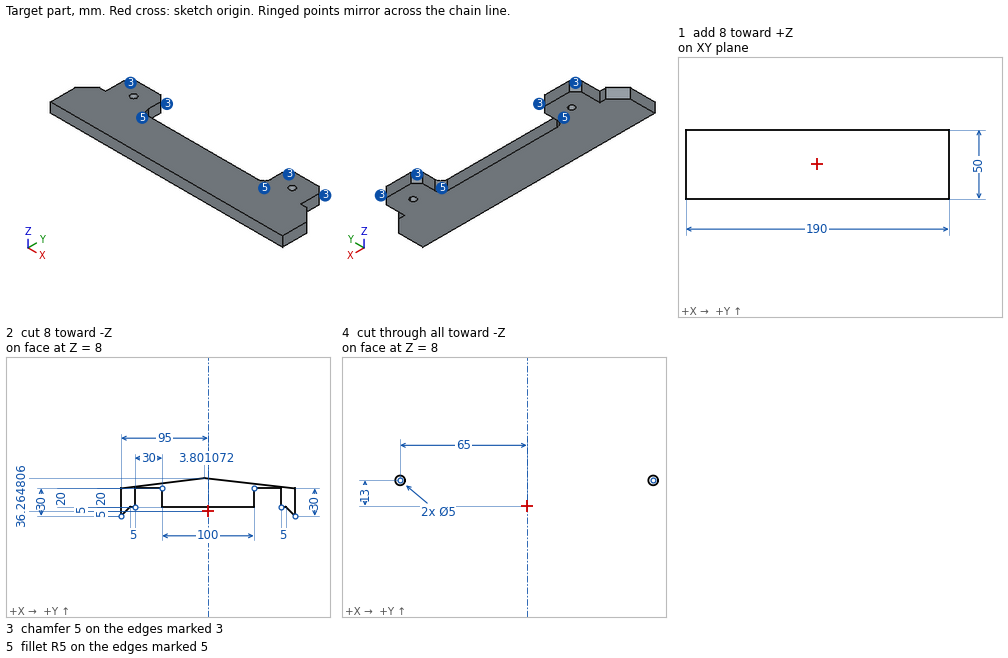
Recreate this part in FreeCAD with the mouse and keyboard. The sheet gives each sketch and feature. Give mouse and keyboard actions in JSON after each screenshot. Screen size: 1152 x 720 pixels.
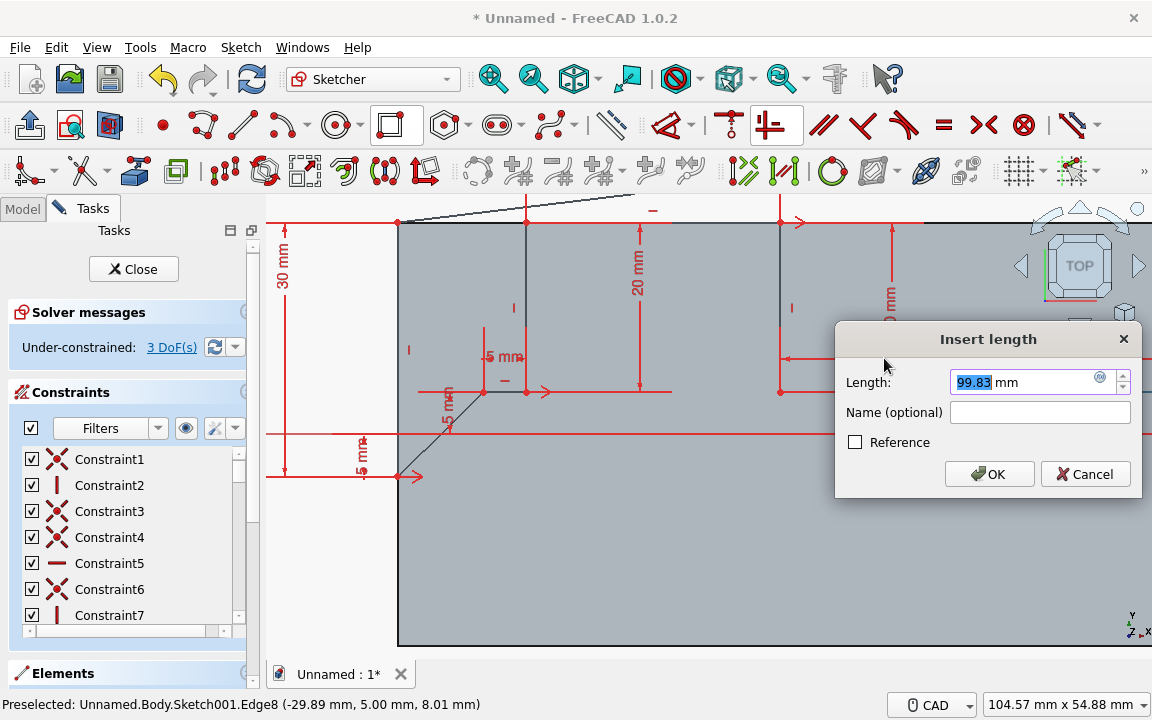
{"action": "type", "text": "100"}
{"action": "key", "text": "Return"}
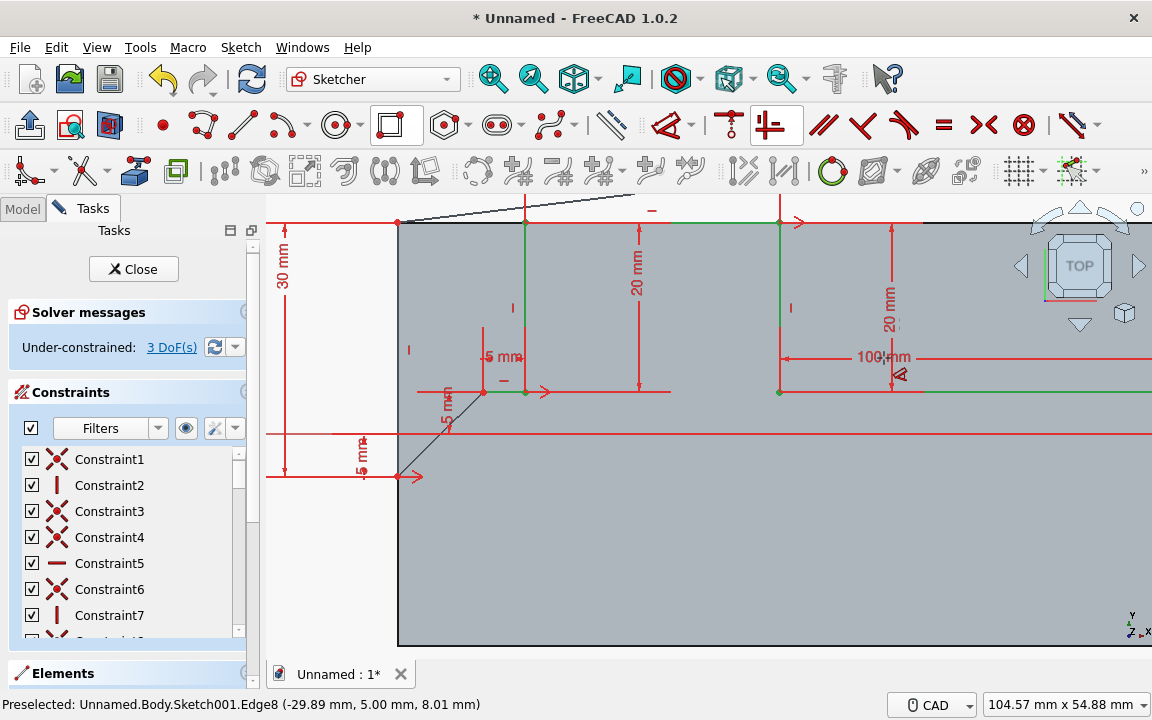
{"action": "left_click", "coordinate": [398, 223]}
{"action": "left_click", "coordinate": [692, 468]}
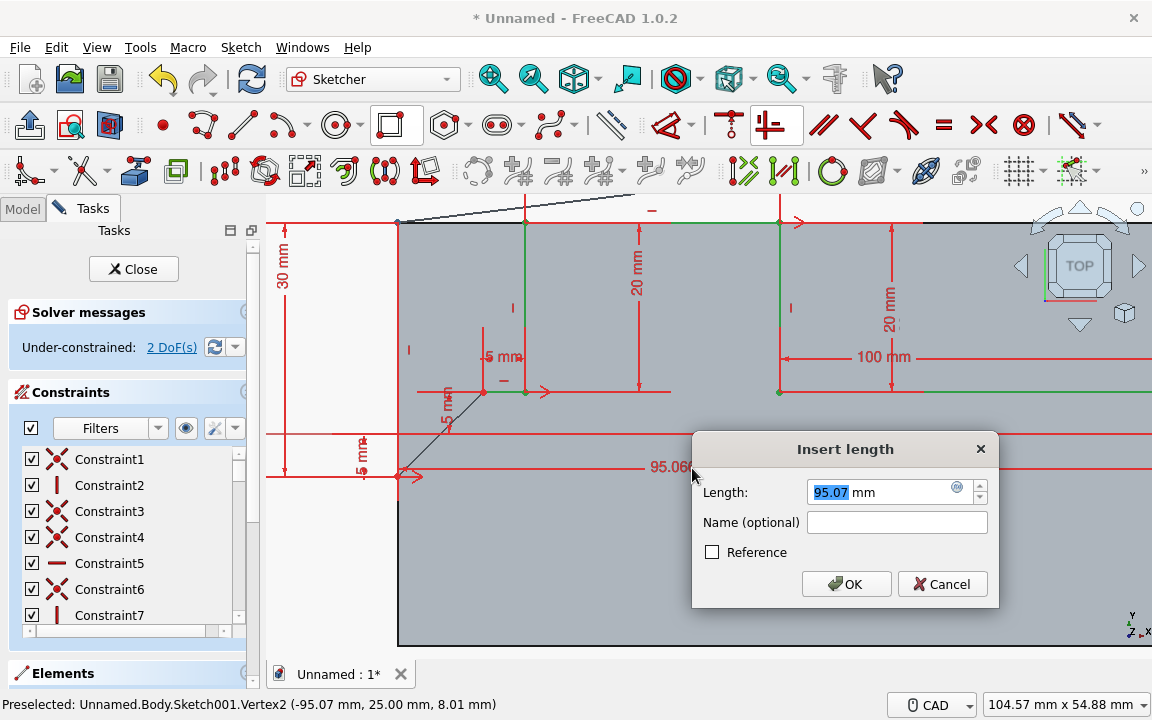
{"action": "type", "text": "95"}
{"action": "key", "text": "Return"}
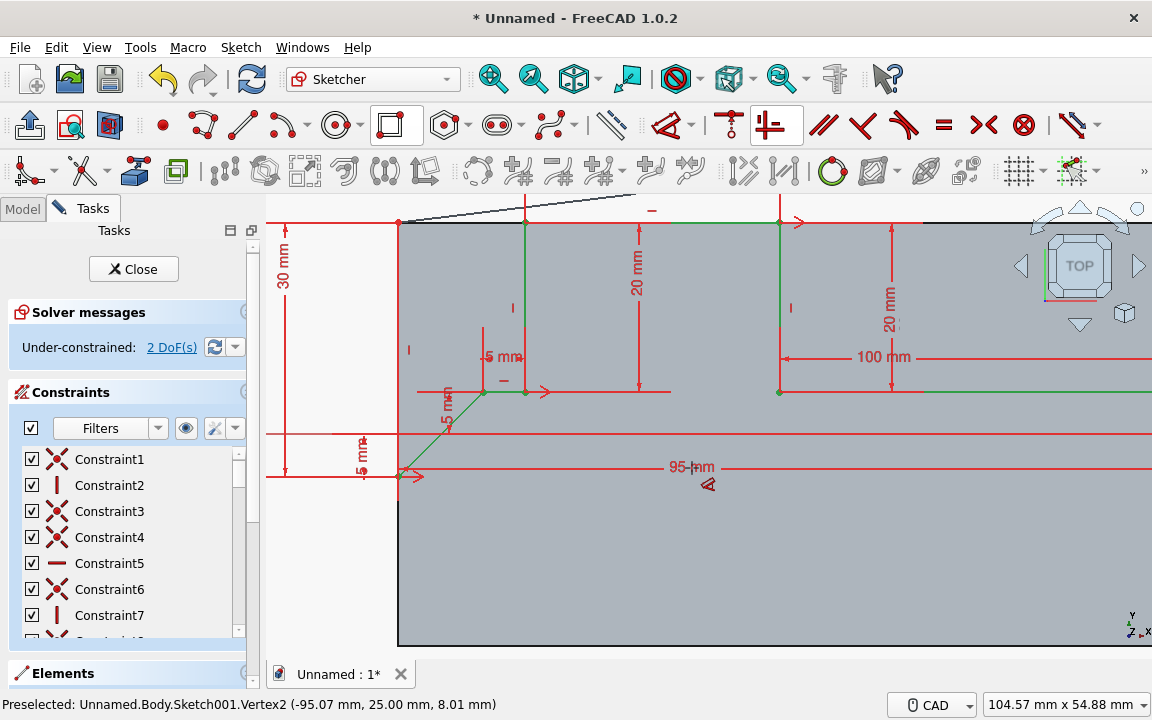
{"action": "scroll", "coordinate": [398, 480], "scroll_direction": "down", "scroll_amount": 6}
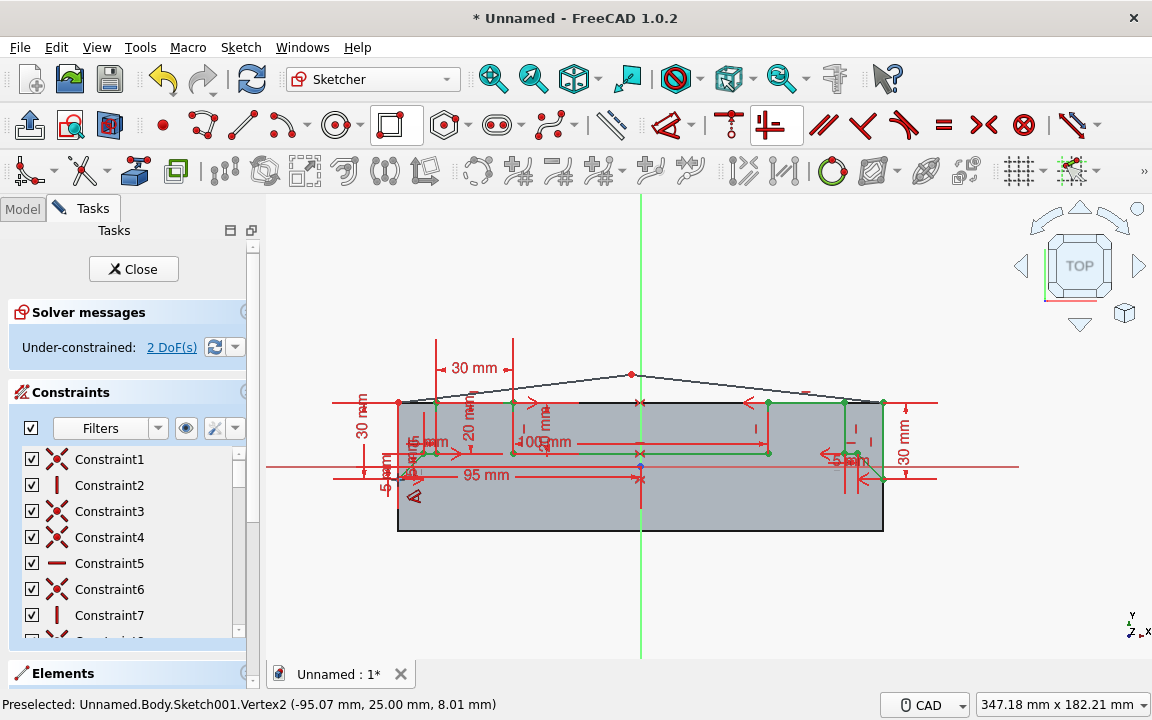
{"action": "scroll", "coordinate": [631, 375], "scroll_direction": "up", "scroll_amount": 8}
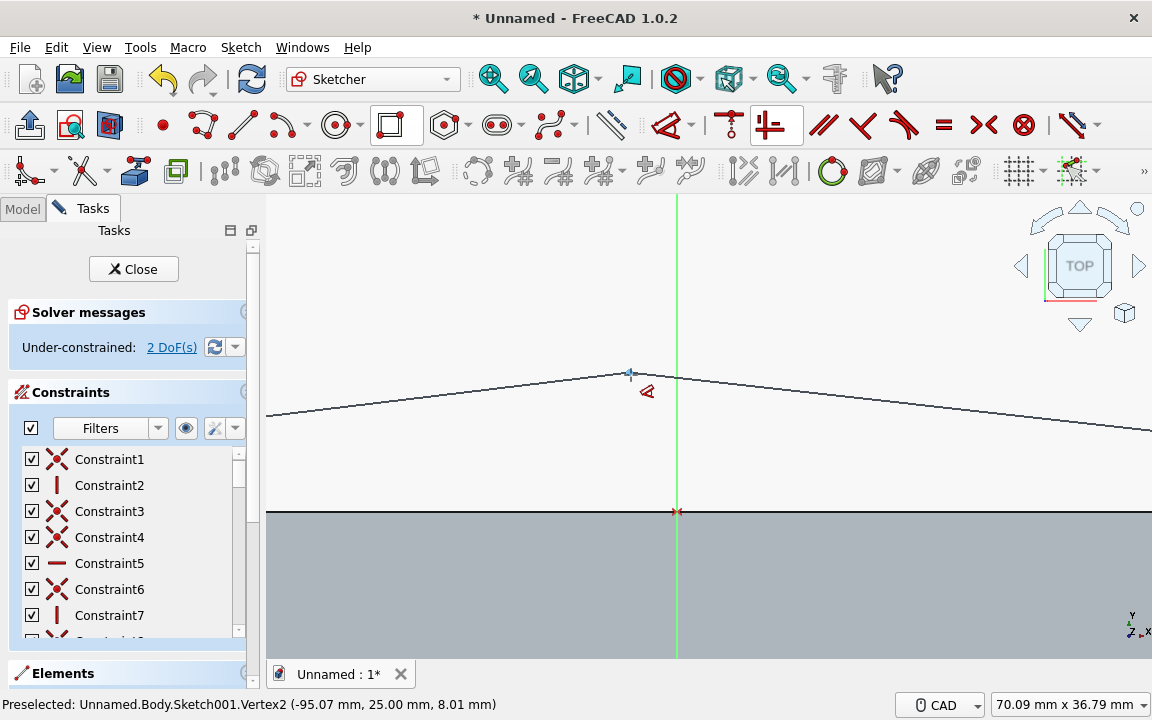
{"action": "left_click", "coordinate": [630, 373]}
{"action": "left_click", "coordinate": [653, 339]}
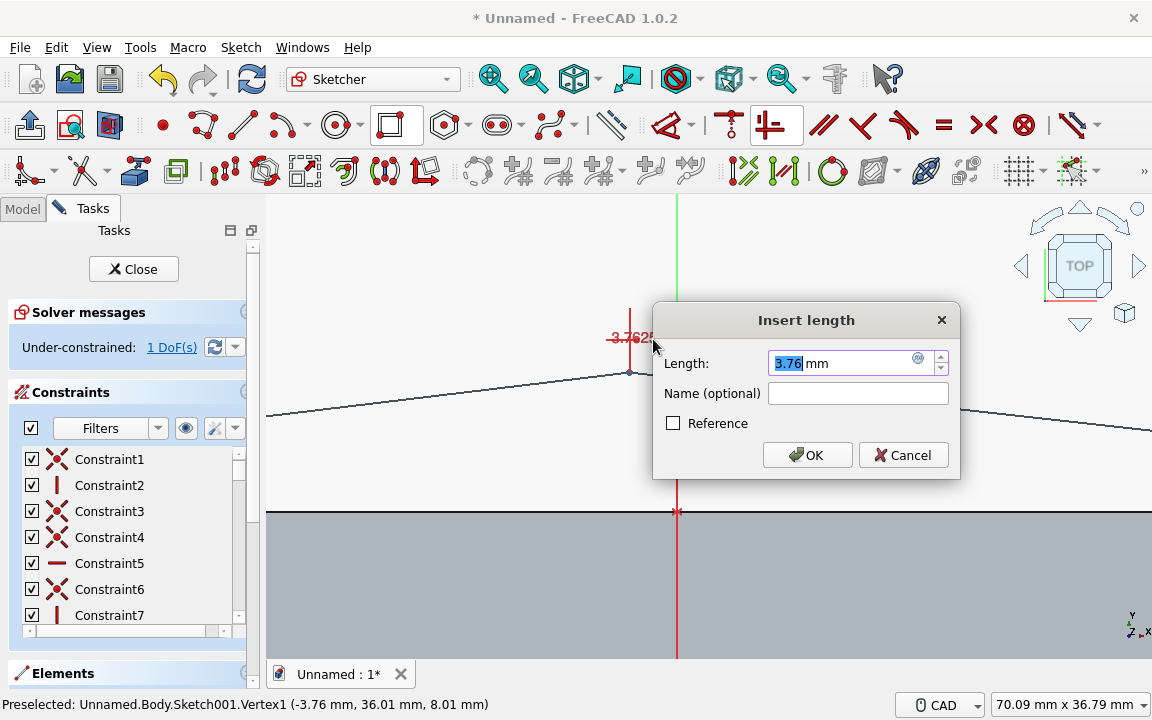
{"action": "type", "text": "3.801072"}
{"action": "key", "text": "Return"}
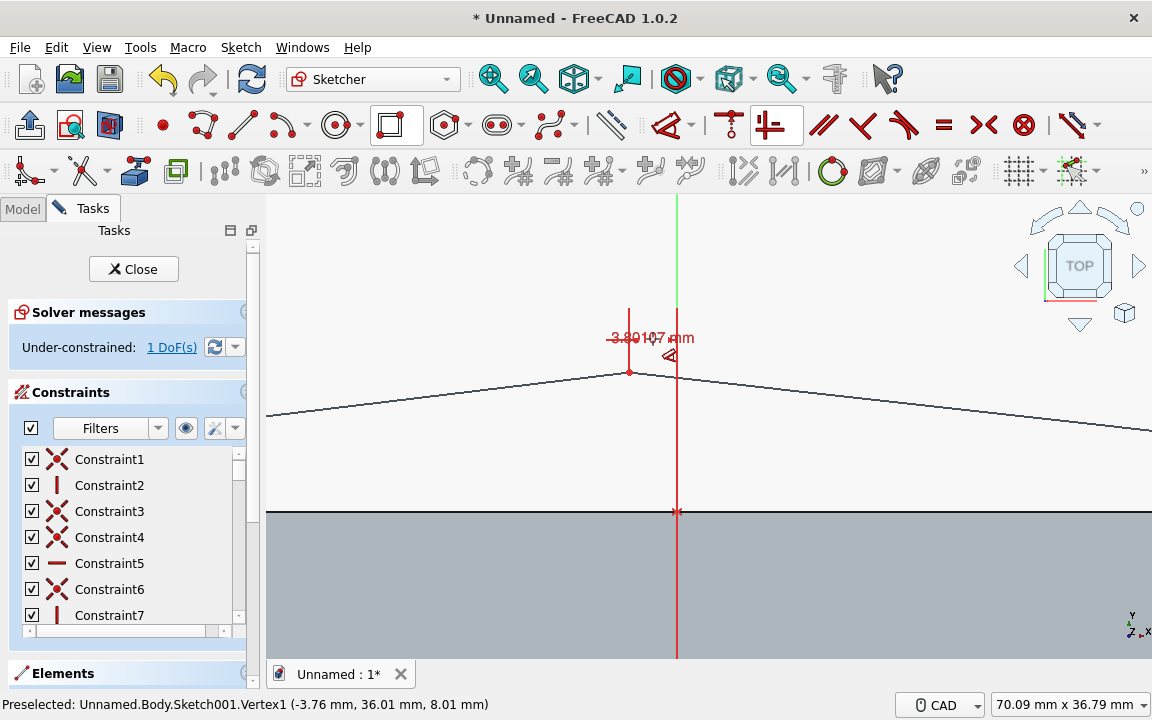
{"action": "scroll", "coordinate": [631, 375], "scroll_direction": "down", "scroll_amount": 8}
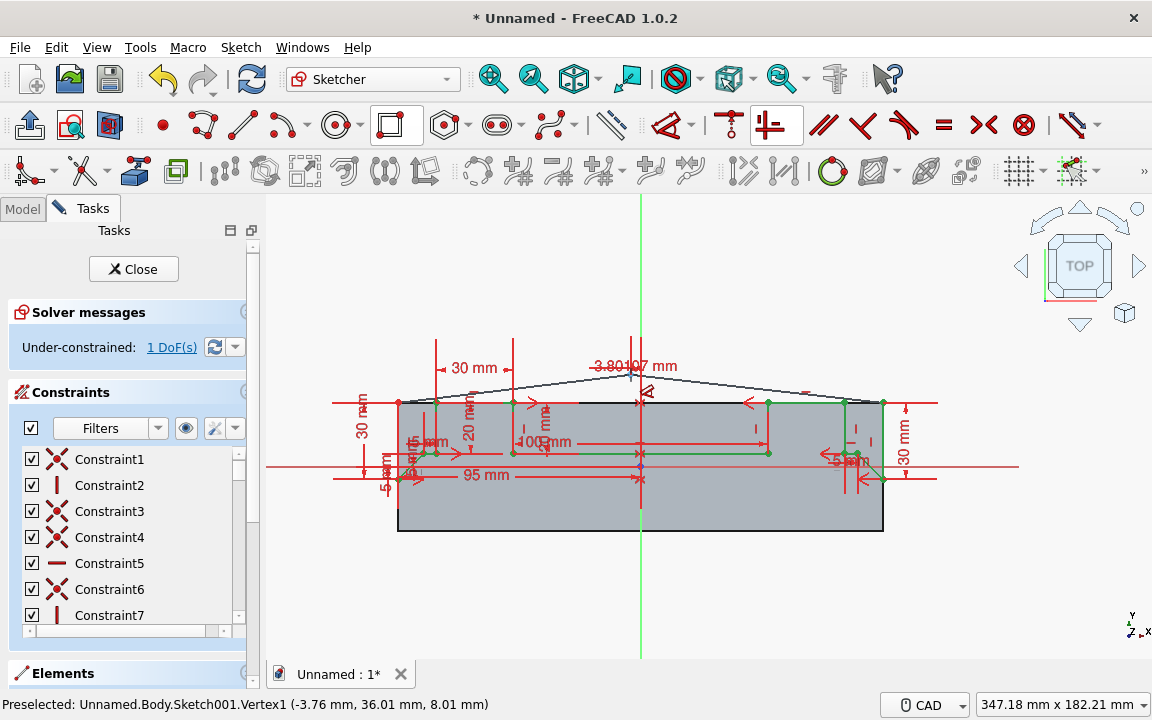
{"action": "left_click", "coordinate": [631, 375]}
{"action": "left_click", "coordinate": [597, 400]}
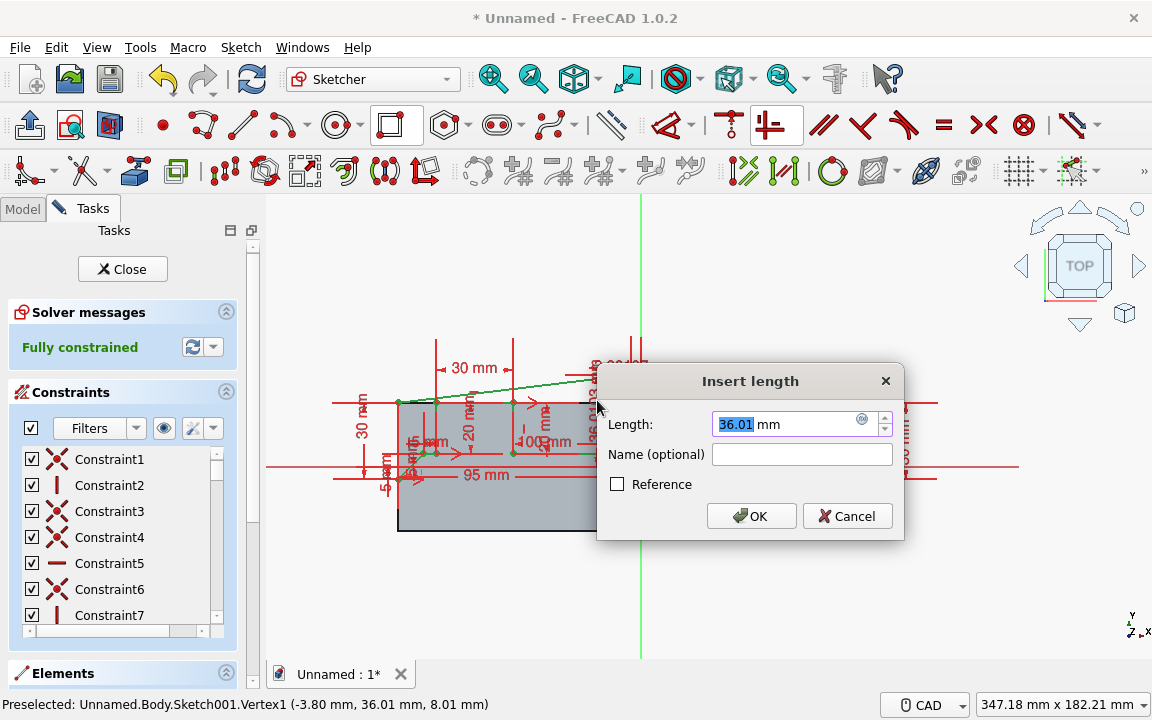
{"action": "type", "text": "36.264806"}
{"action": "key", "text": "Return"}
{"action": "key", "text": "Escape"}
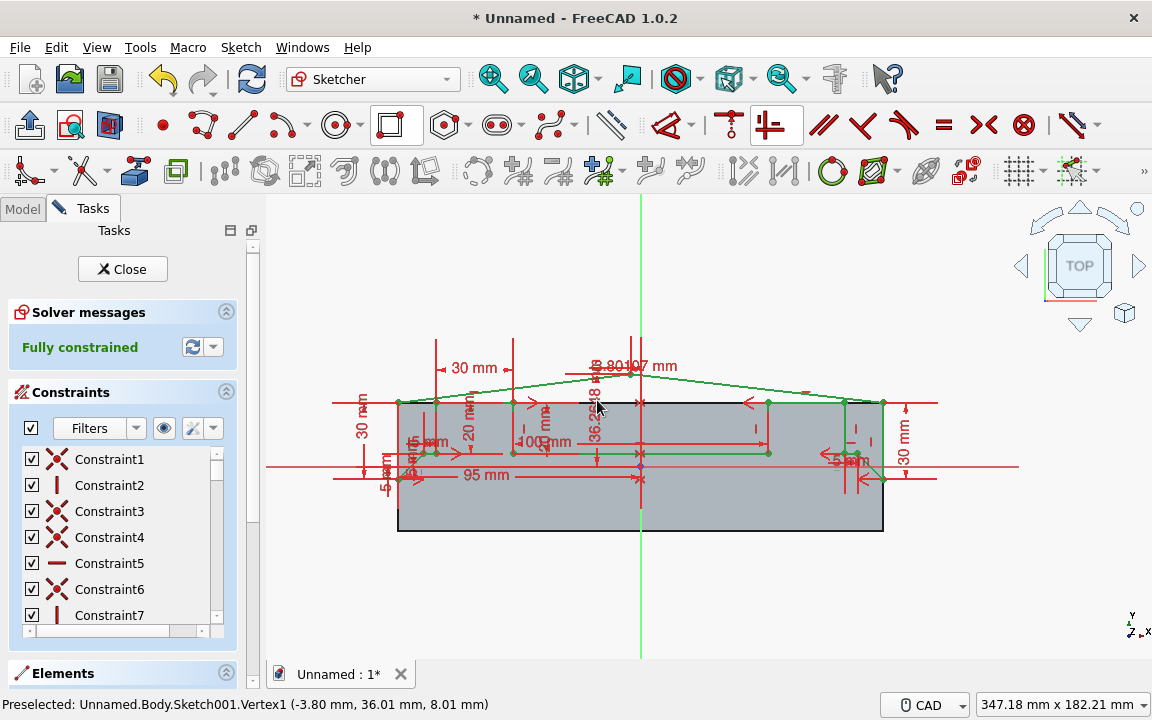
{"action": "left_click", "coordinate": [123, 269]}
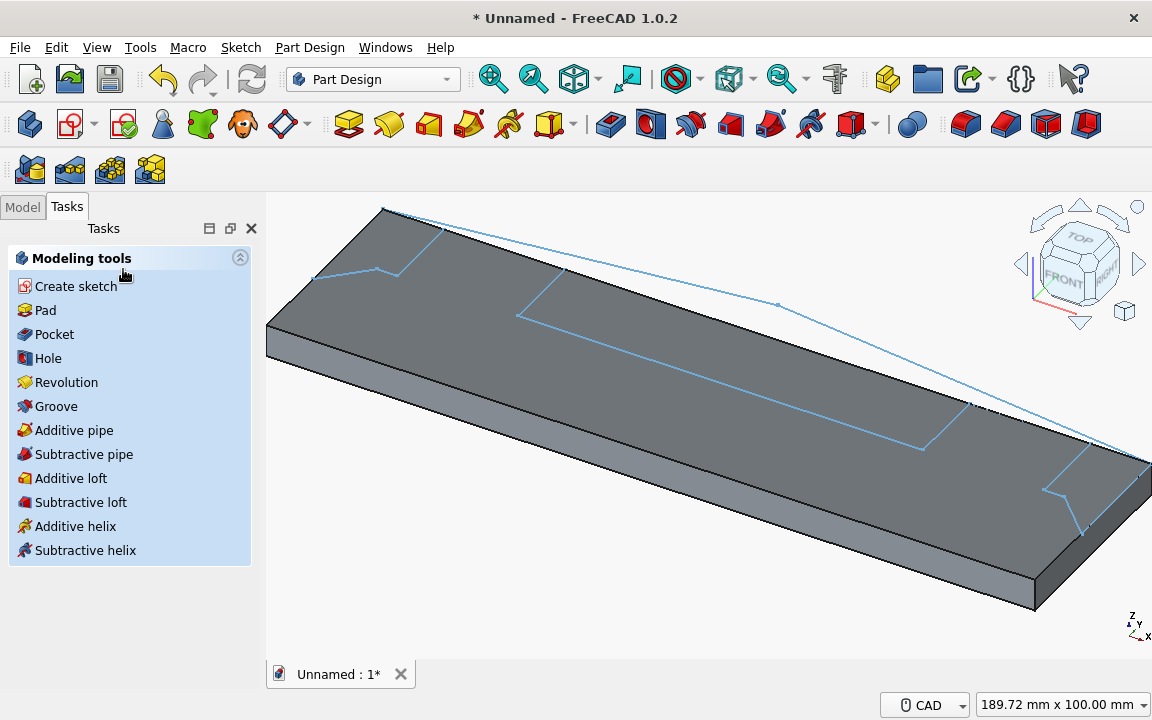
{"action": "left_click", "coordinate": [612, 124]}